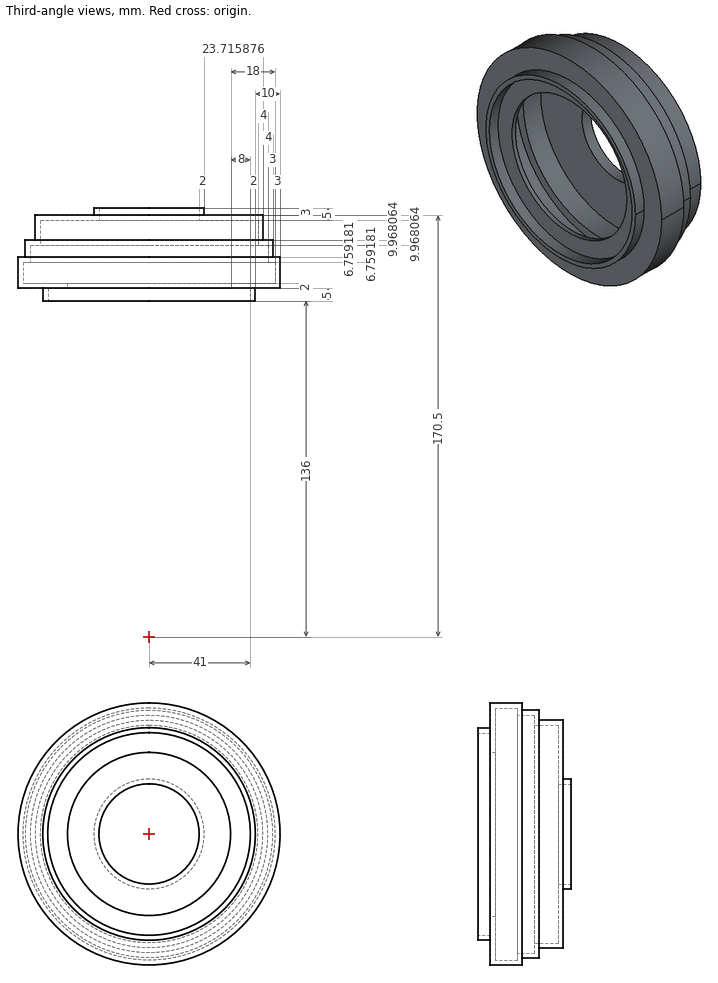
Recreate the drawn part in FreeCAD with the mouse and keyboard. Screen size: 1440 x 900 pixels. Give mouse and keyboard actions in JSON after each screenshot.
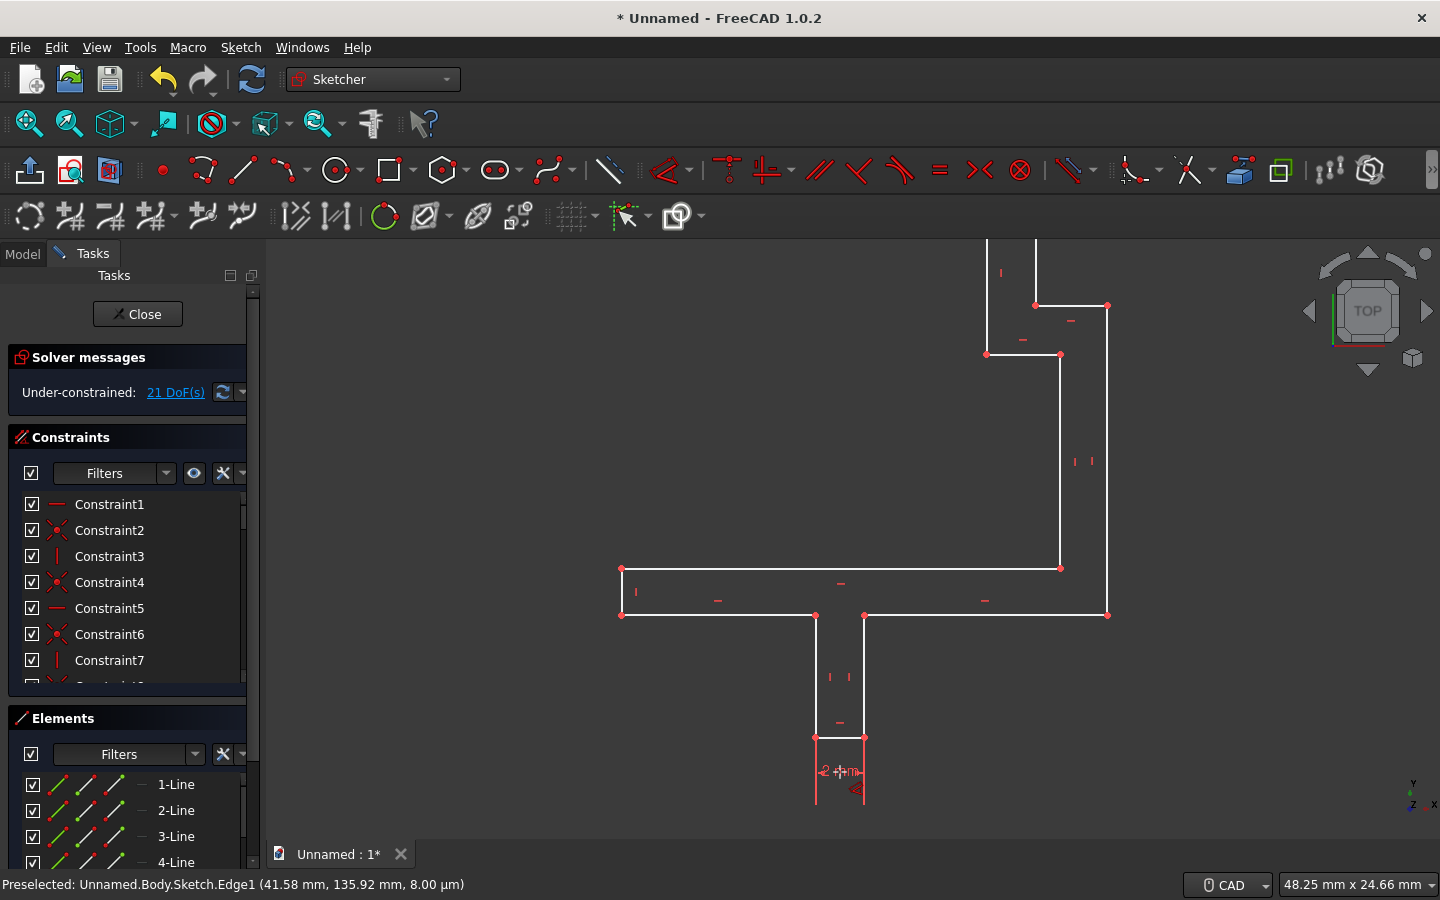
{"action": "left_click", "coordinate": [864, 701]}
{"action": "left_click", "coordinate": [898, 677]}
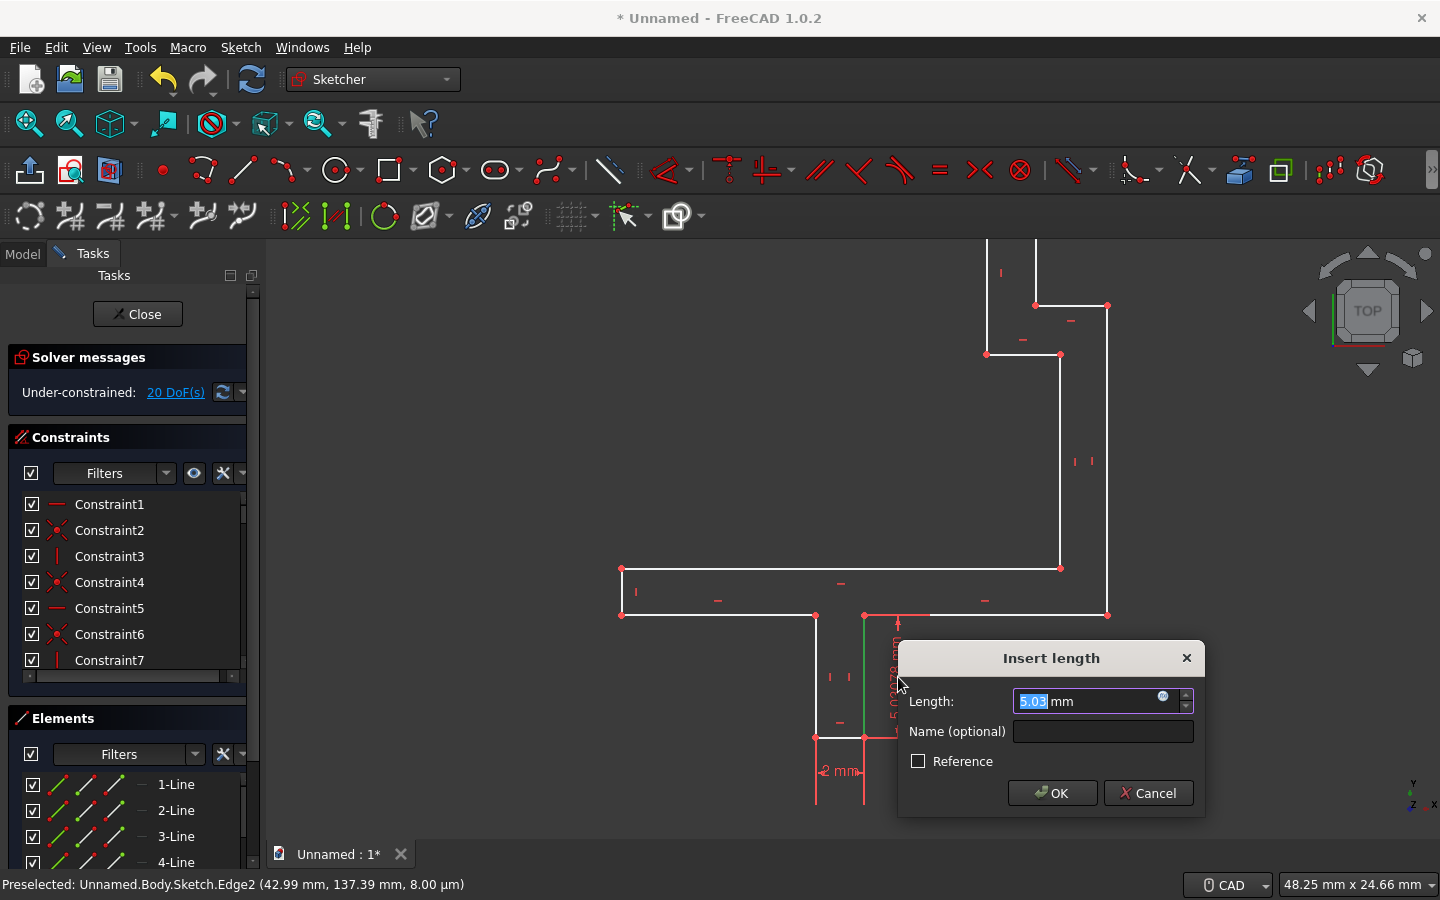
{"action": "type", "text": "5"}
{"action": "key", "text": "Return"}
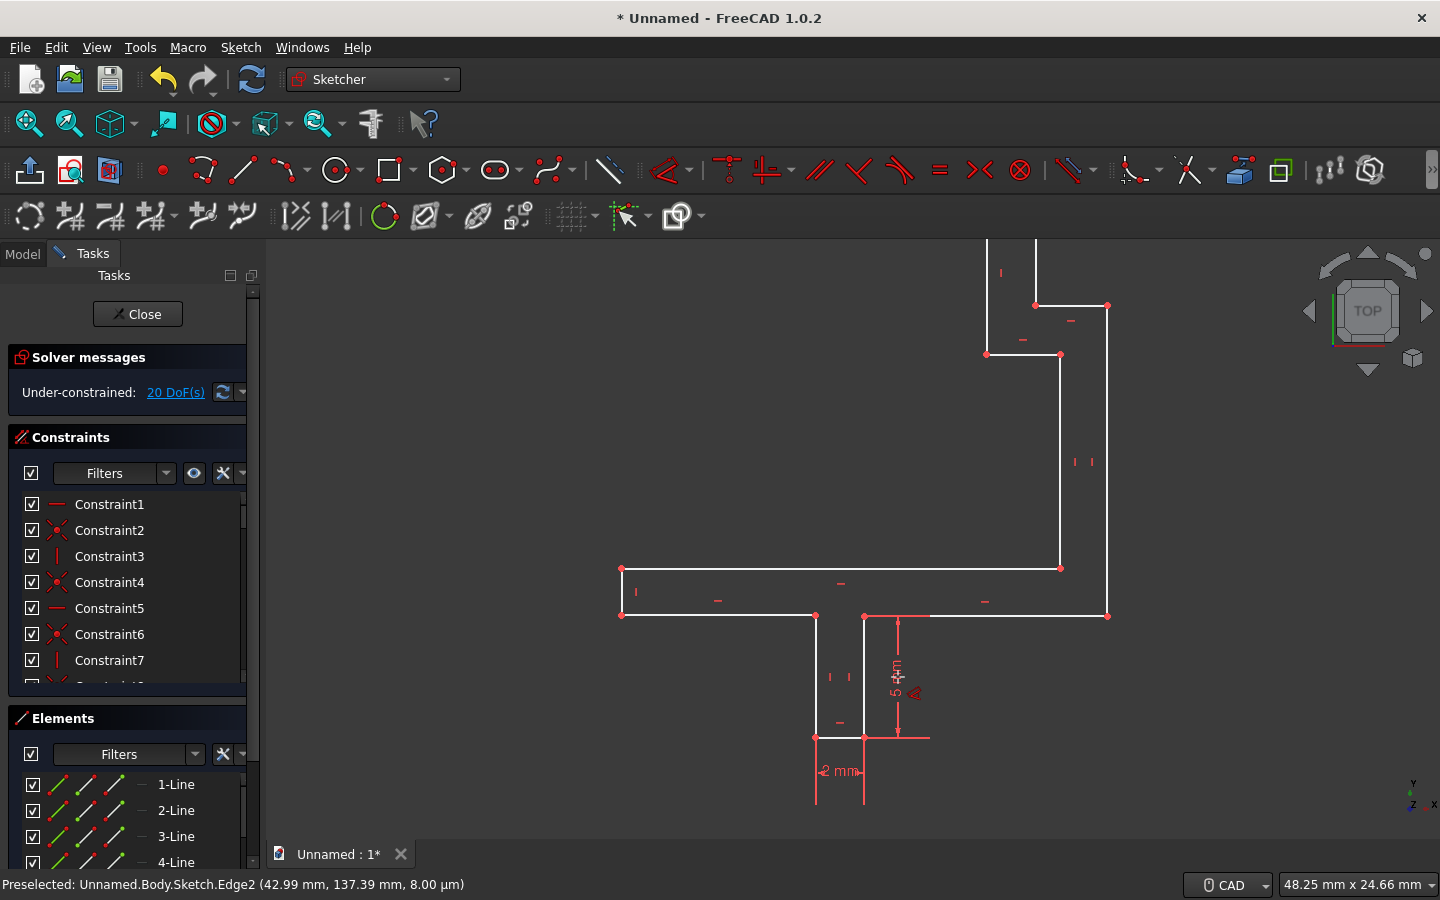
{"action": "left_click", "coordinate": [1086, 306]}
{"action": "left_click", "coordinate": [1071, 340]}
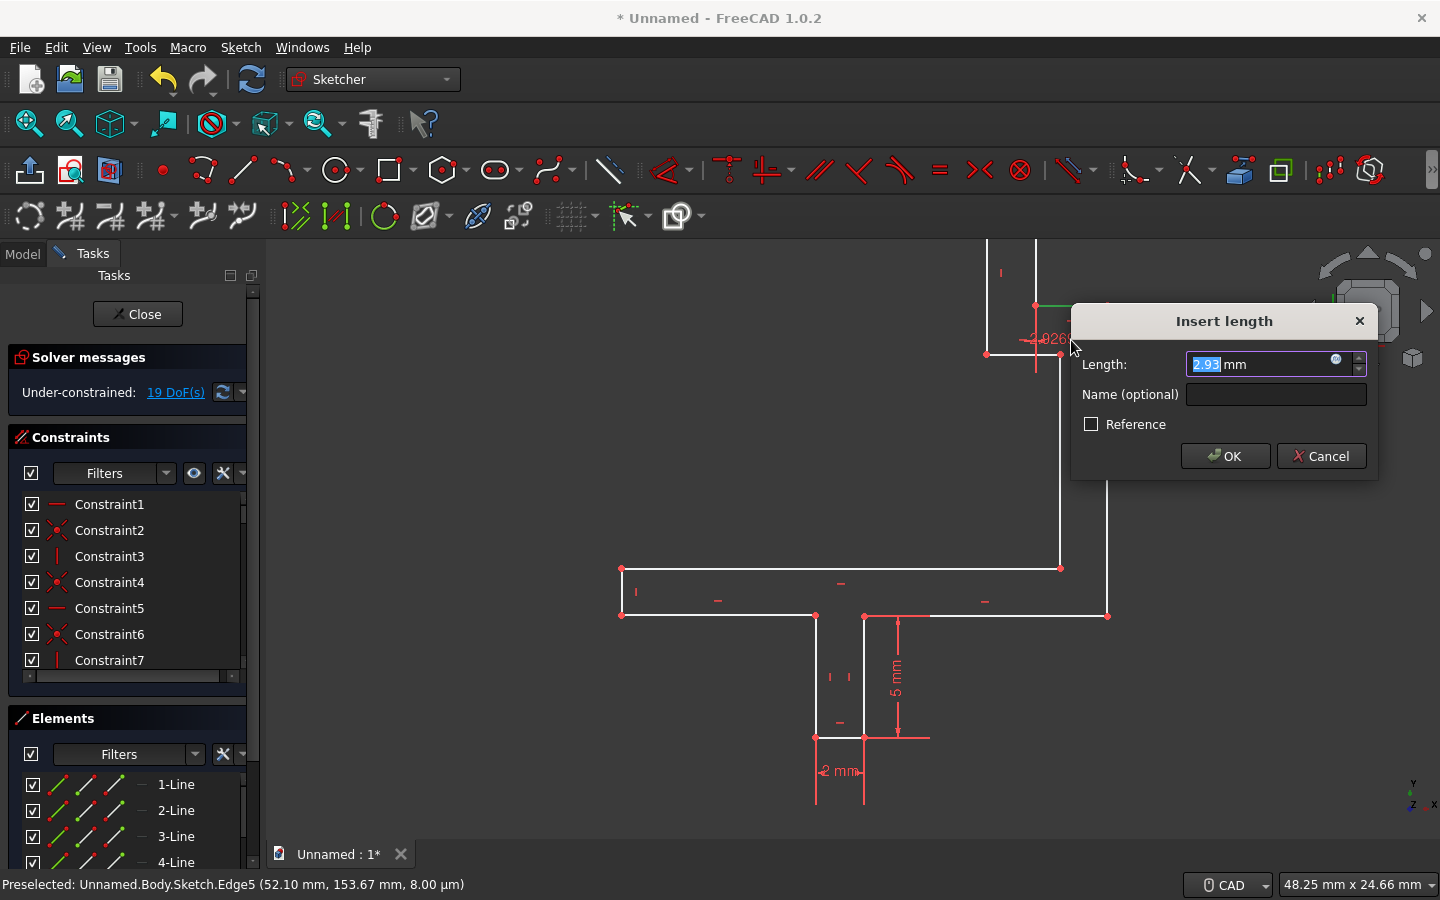
{"action": "type", "text": "3"}
{"action": "key", "text": "Return"}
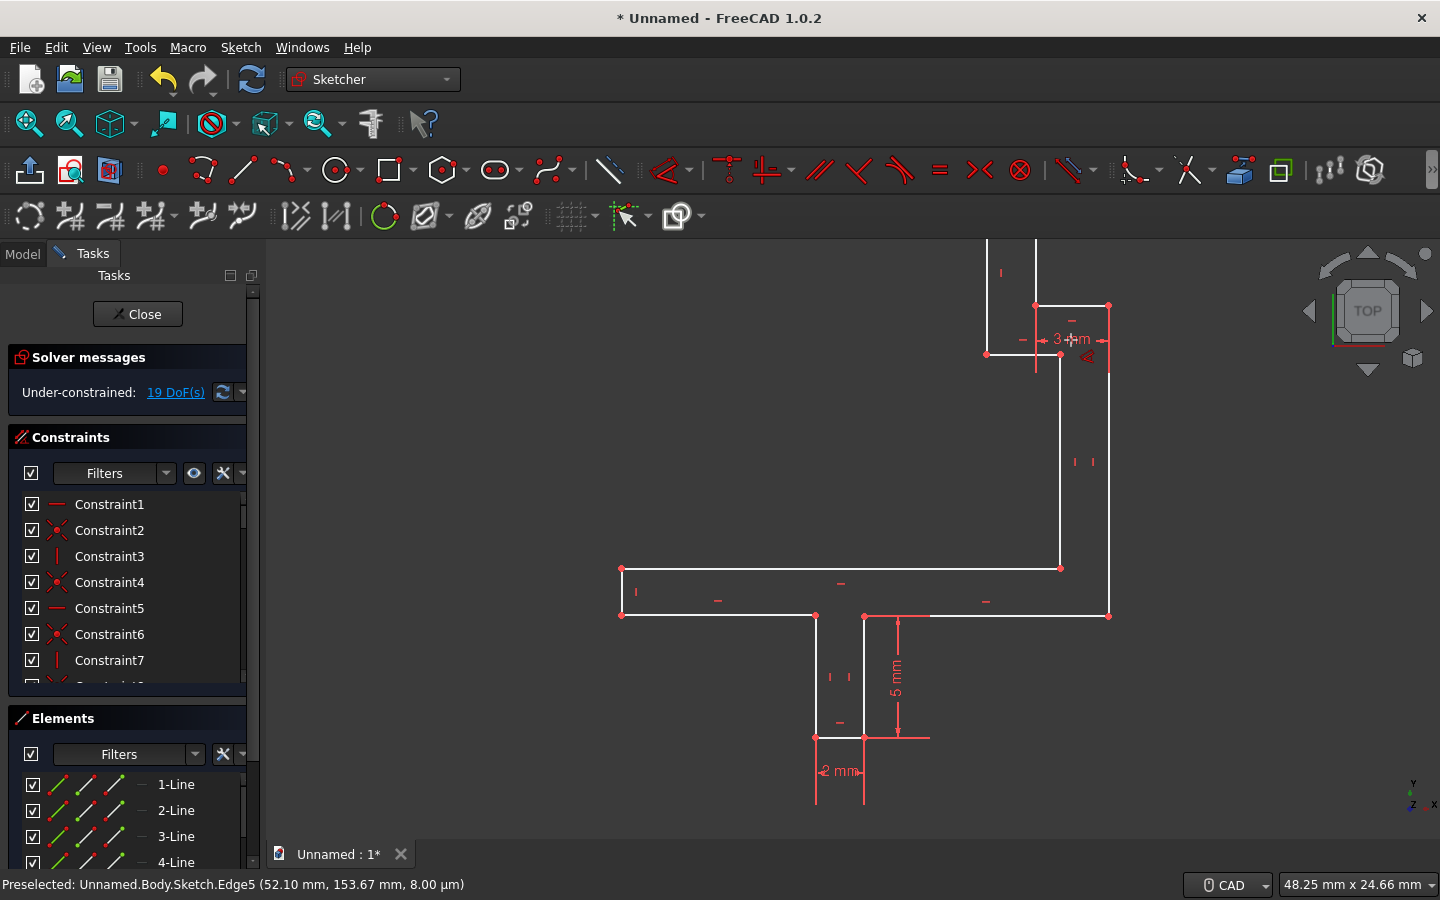
{"action": "scroll", "coordinate": [845, 751], "scroll_direction": "down", "scroll_amount": 4}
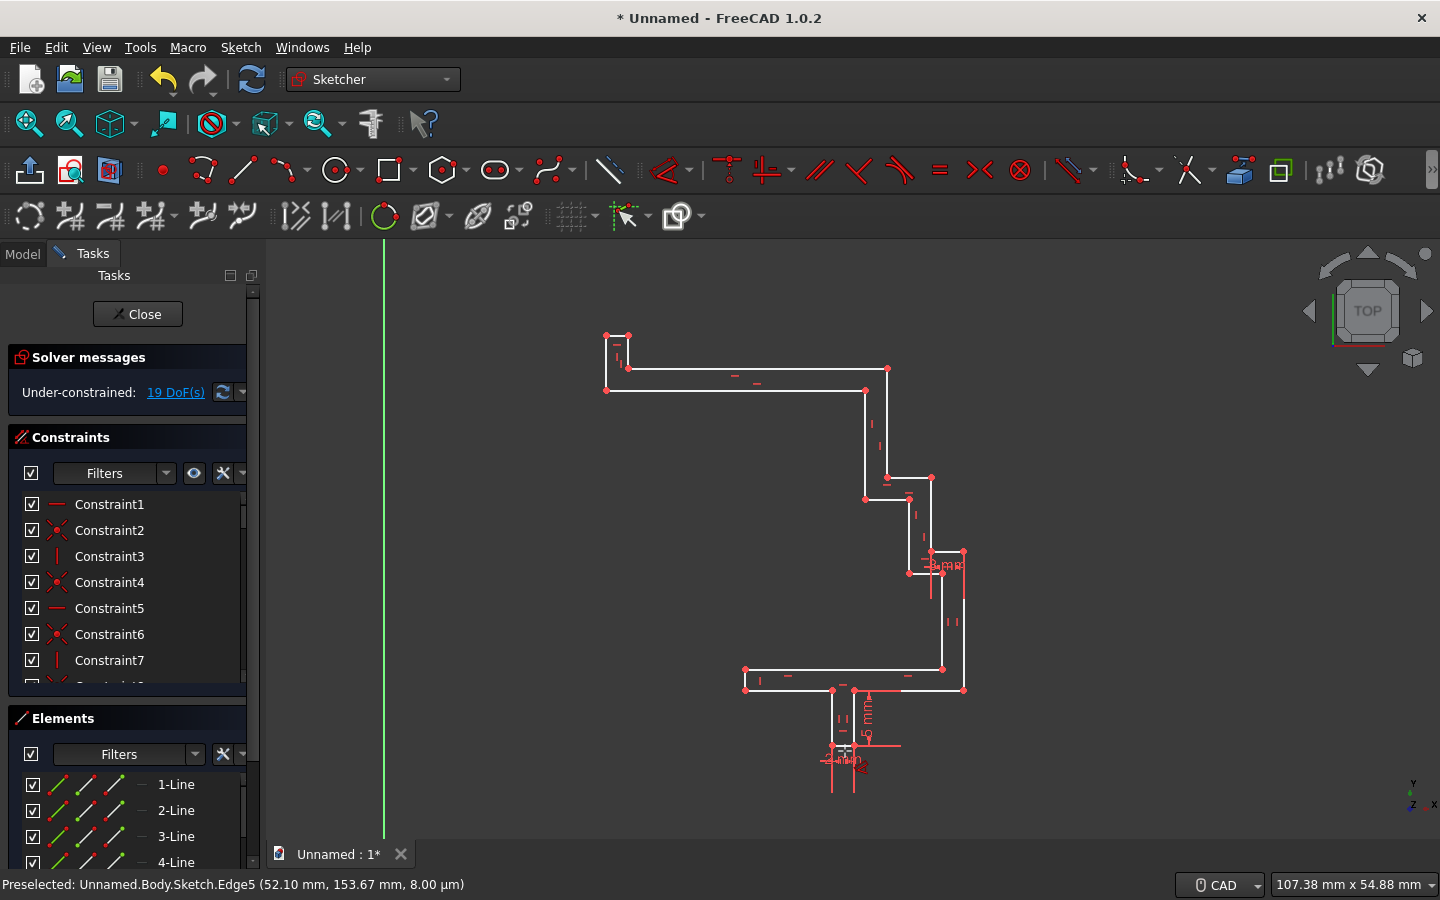
{"action": "left_click", "coordinate": [918, 478]}
{"action": "left_click", "coordinate": [909, 444]}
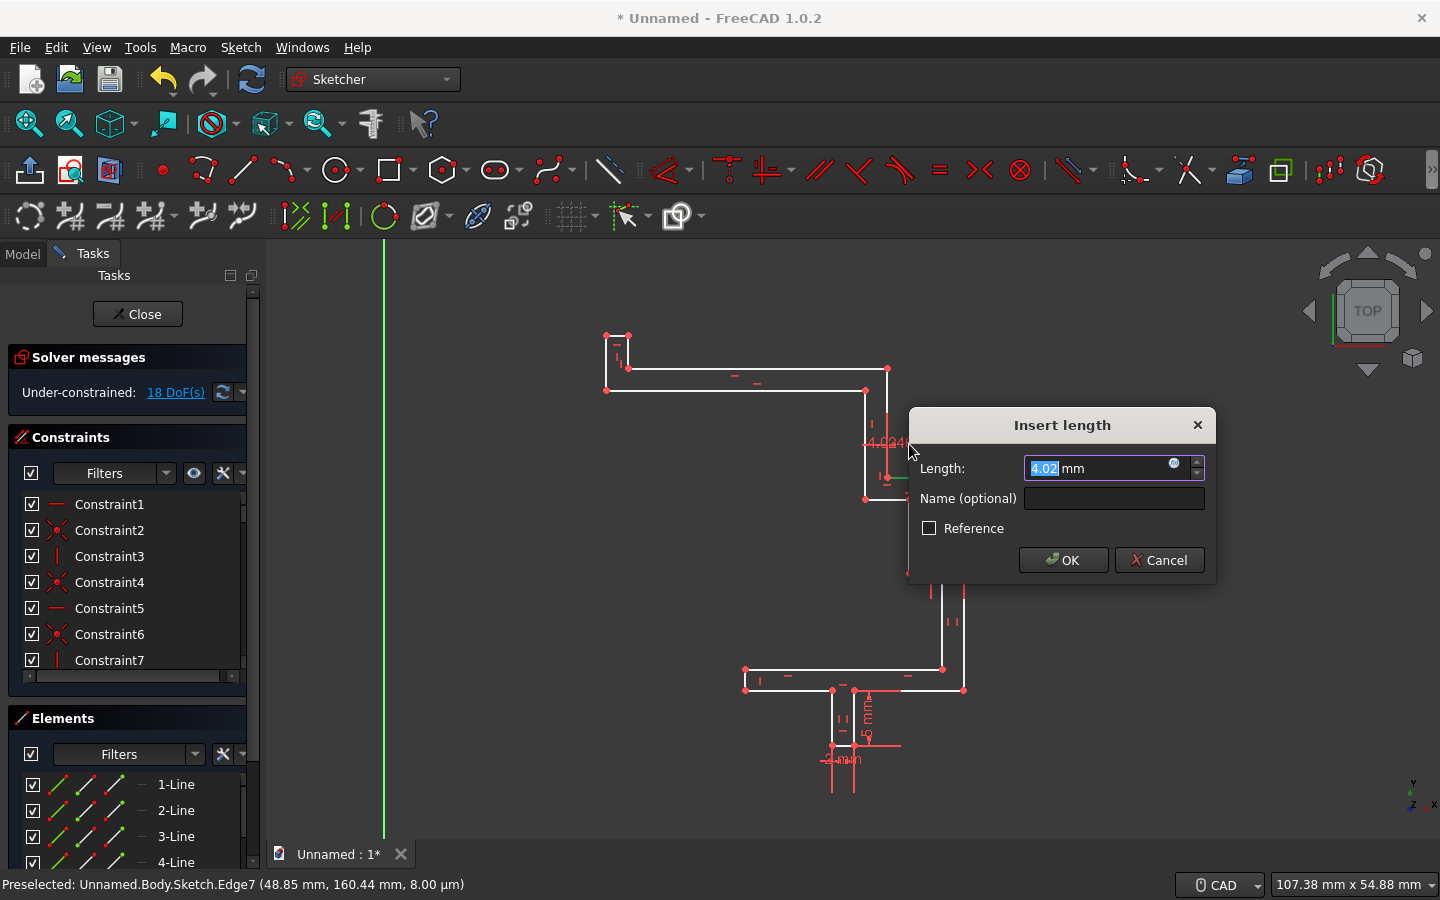
{"action": "type", "text": "4"}
{"action": "key", "text": "Return"}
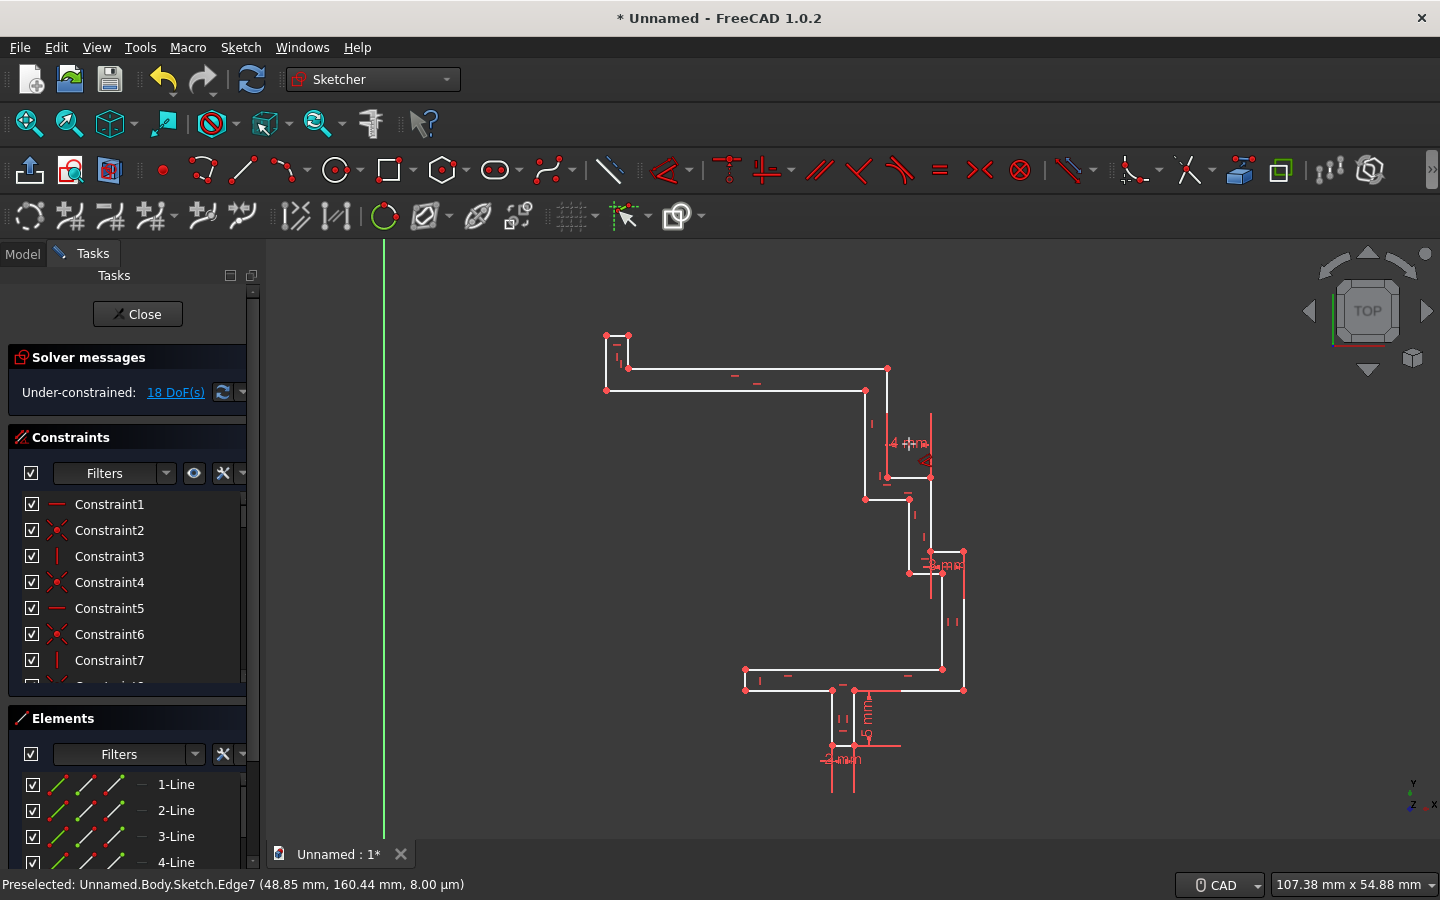
{"action": "scroll", "coordinate": [628, 359], "scroll_direction": "up", "scroll_amount": 2}